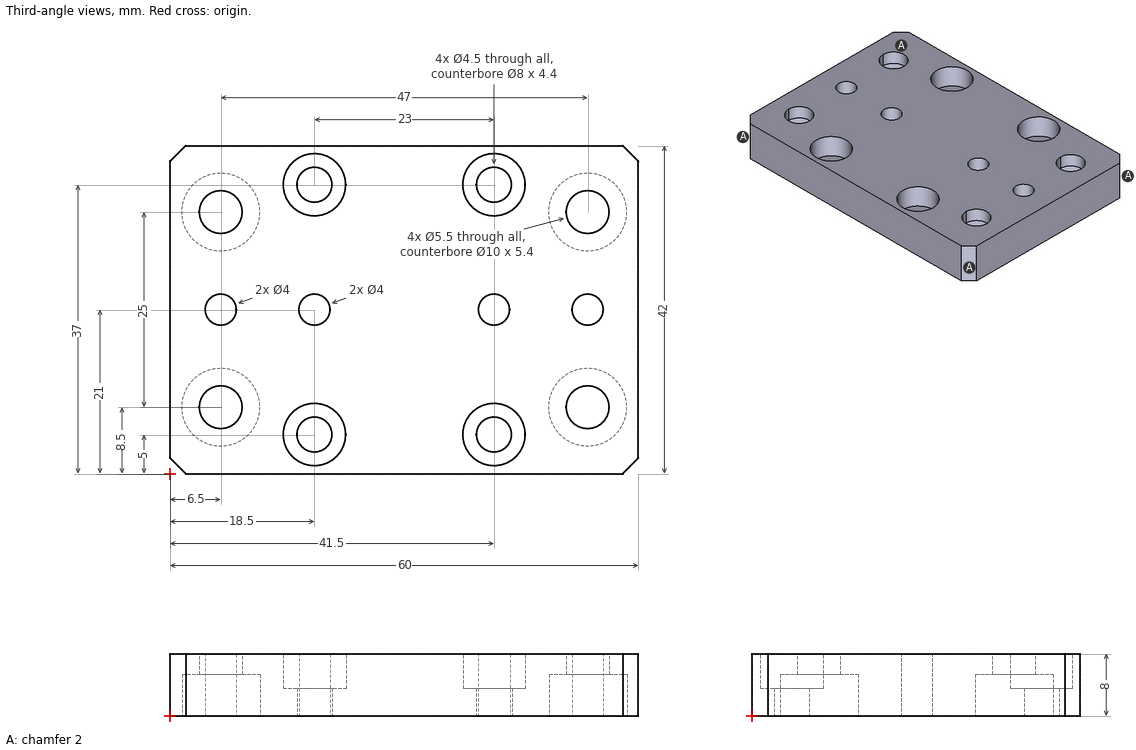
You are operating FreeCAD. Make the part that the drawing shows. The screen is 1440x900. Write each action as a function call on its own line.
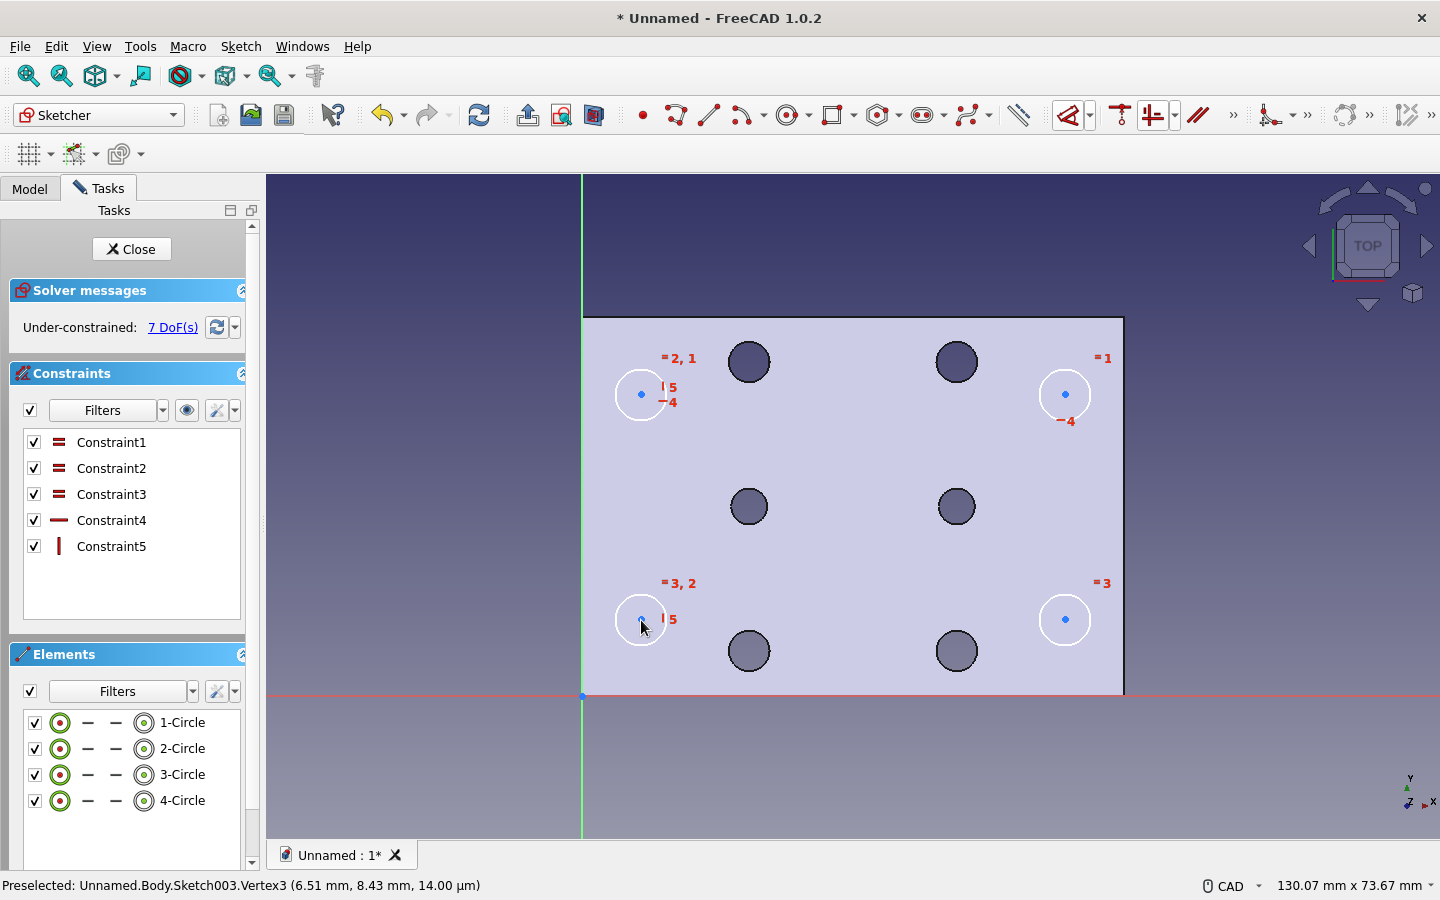
click(1065, 395)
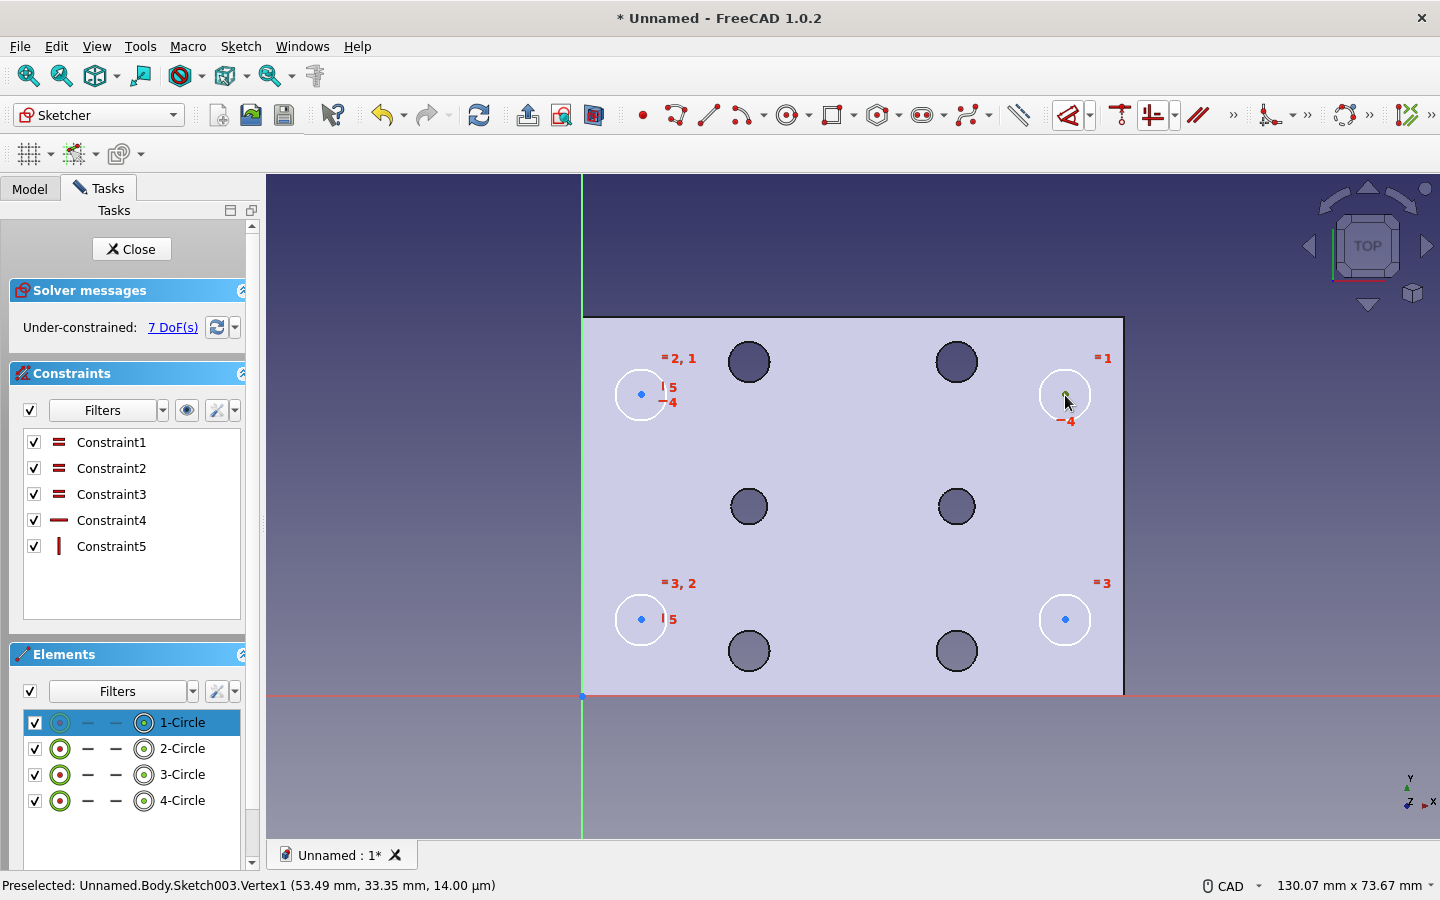
click(1065, 620)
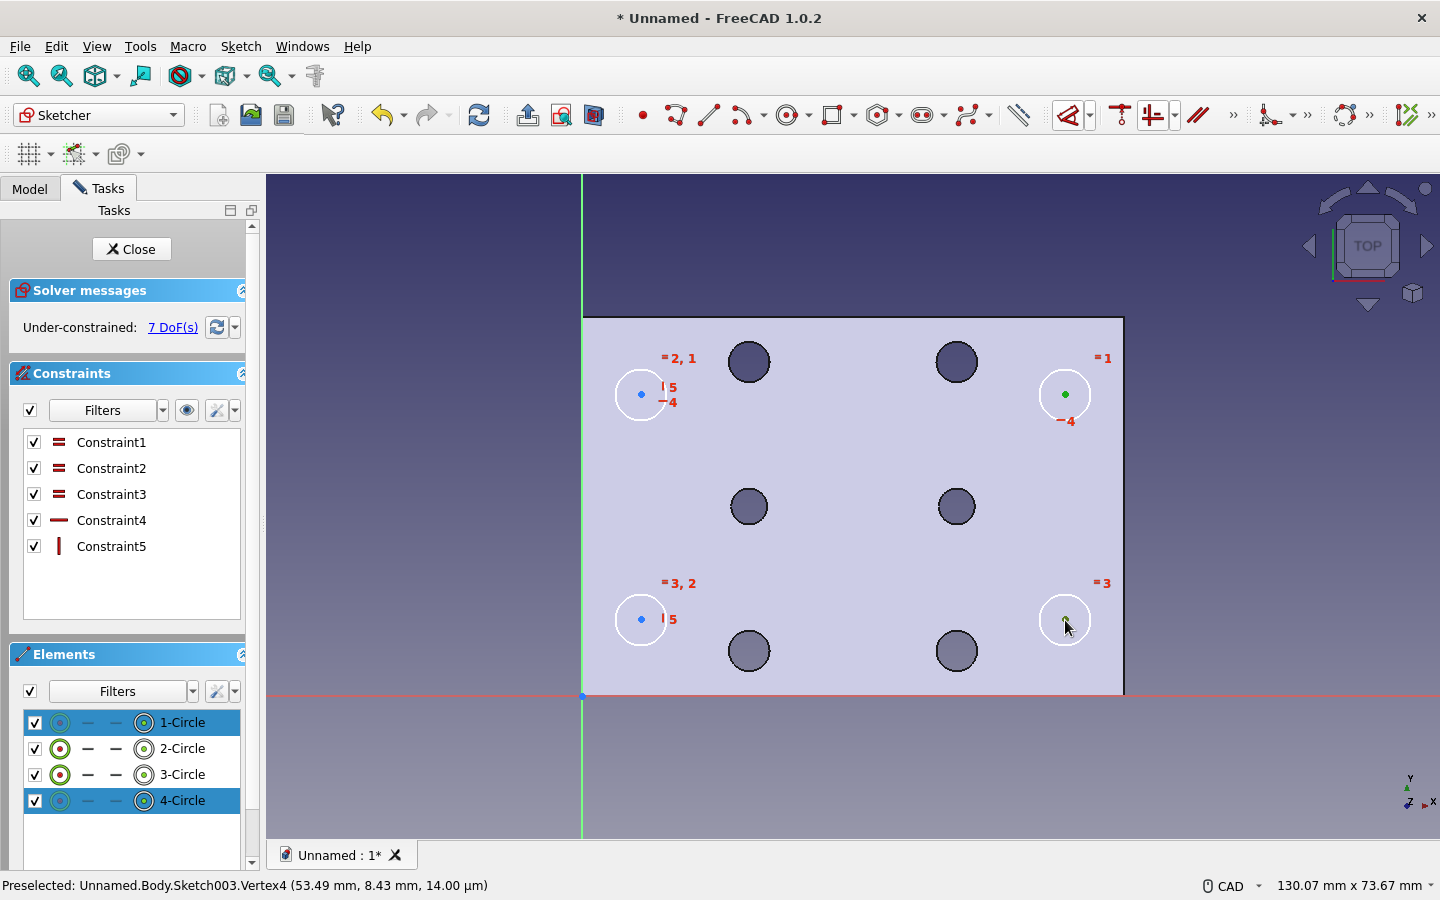
key(v)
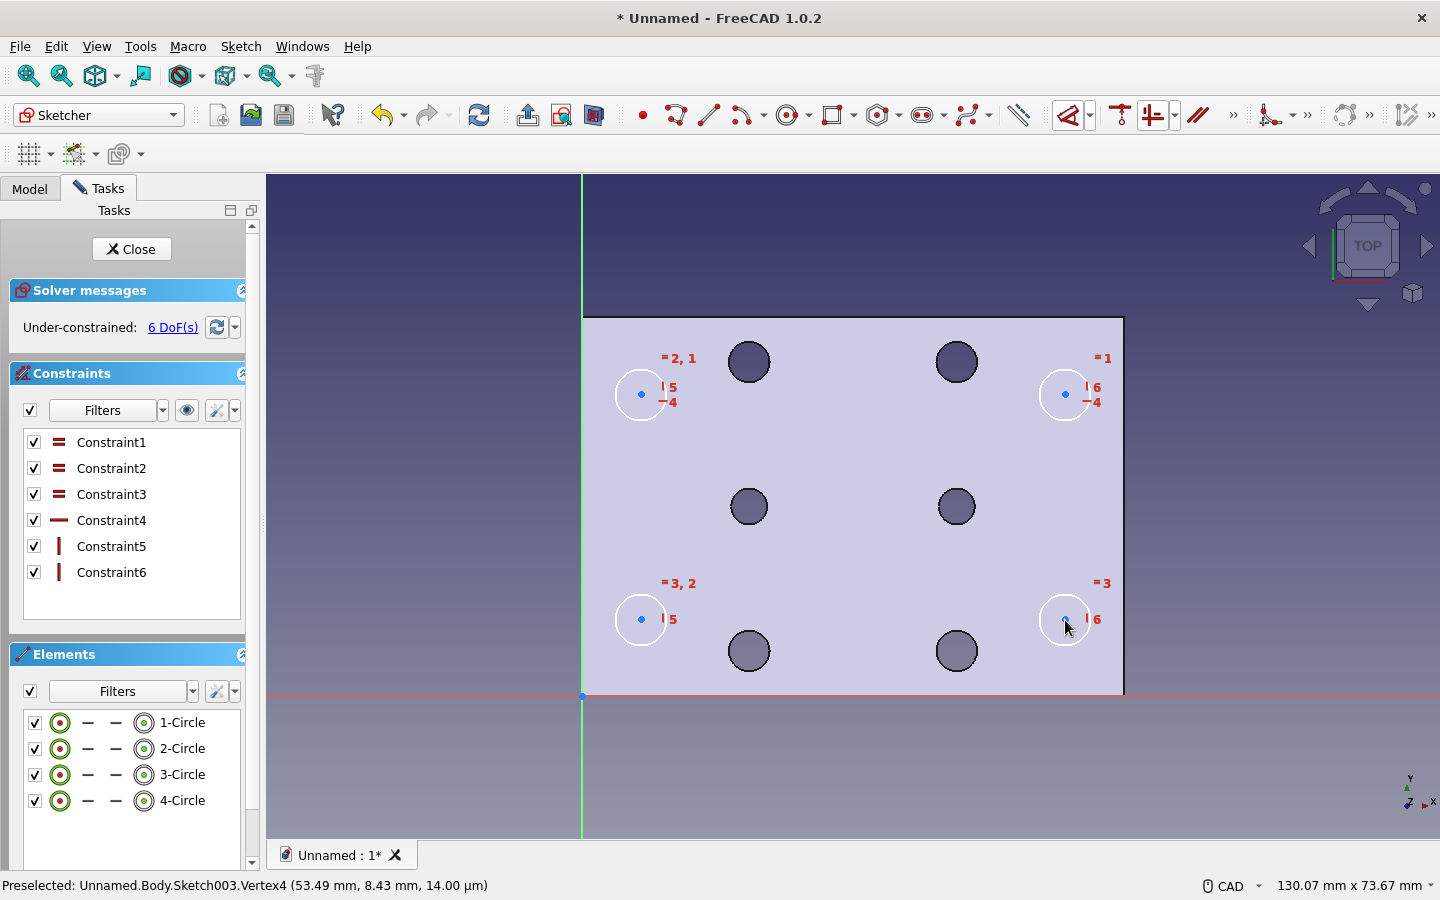
click(641, 620)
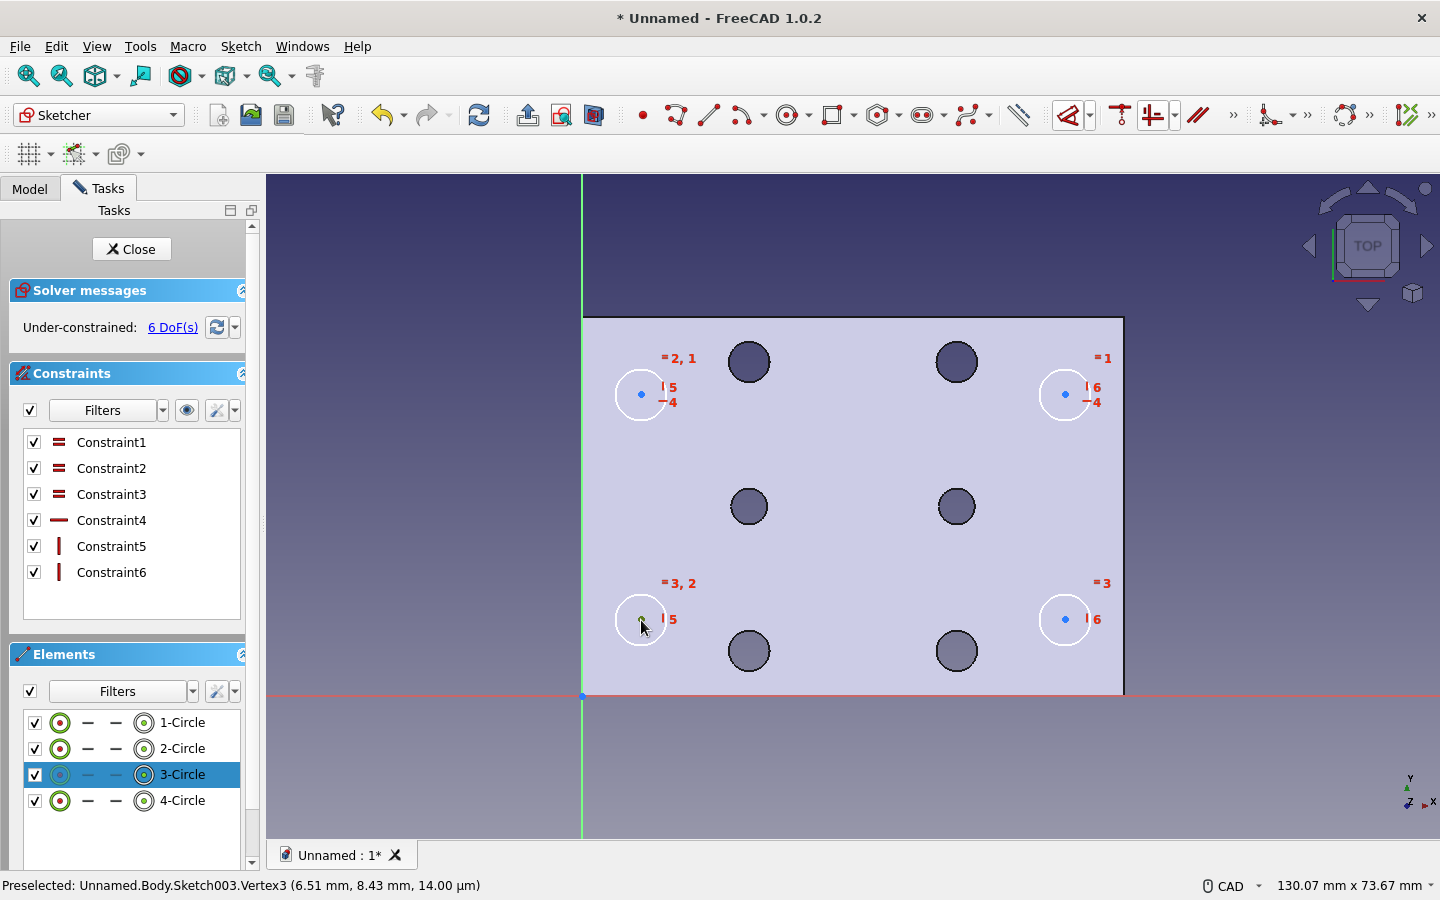
click(1065, 620)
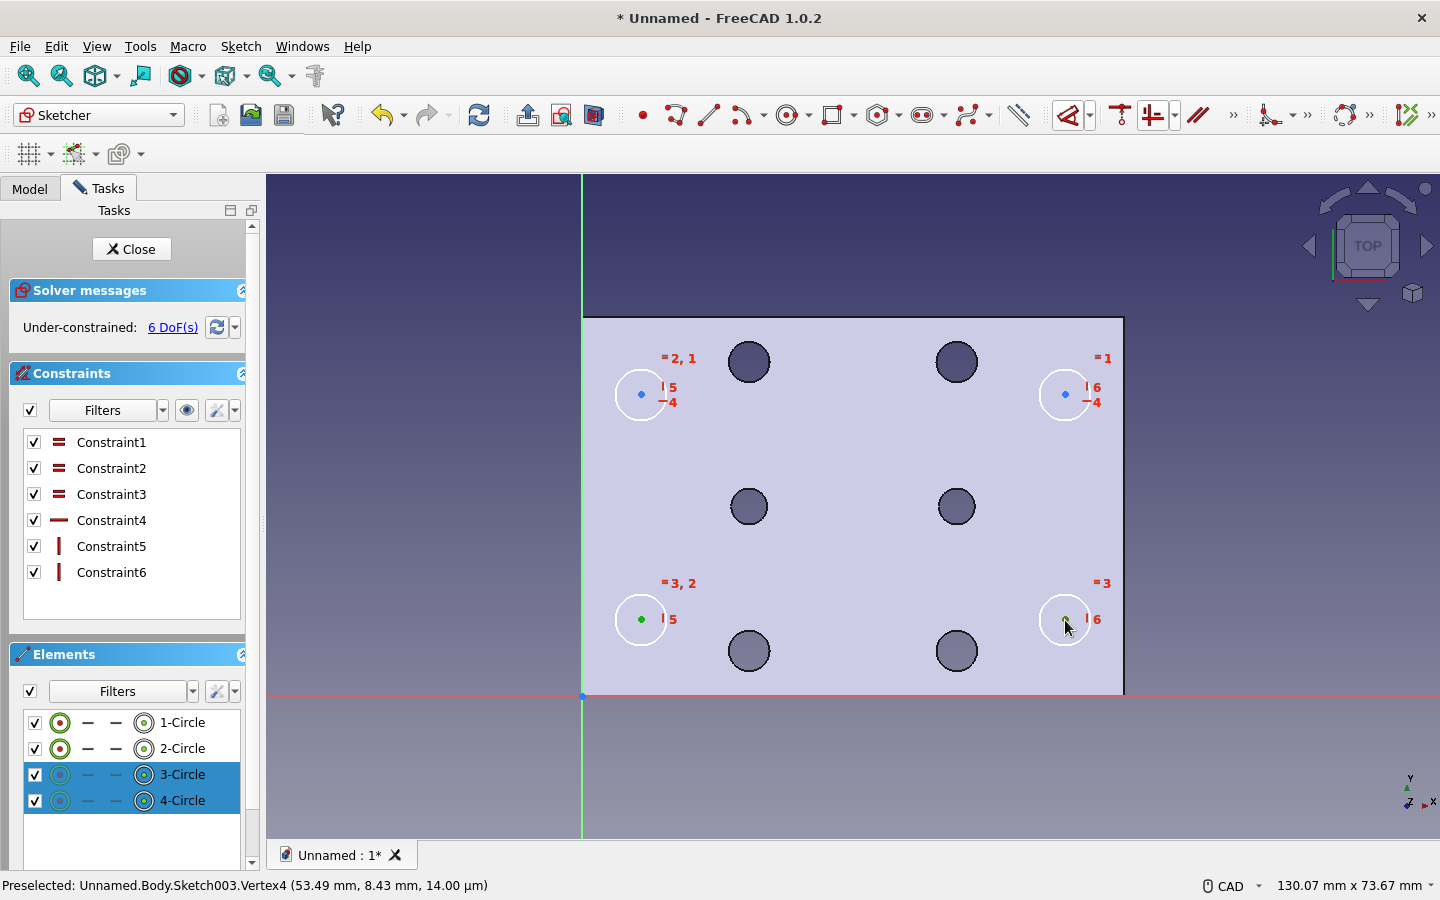
key(h)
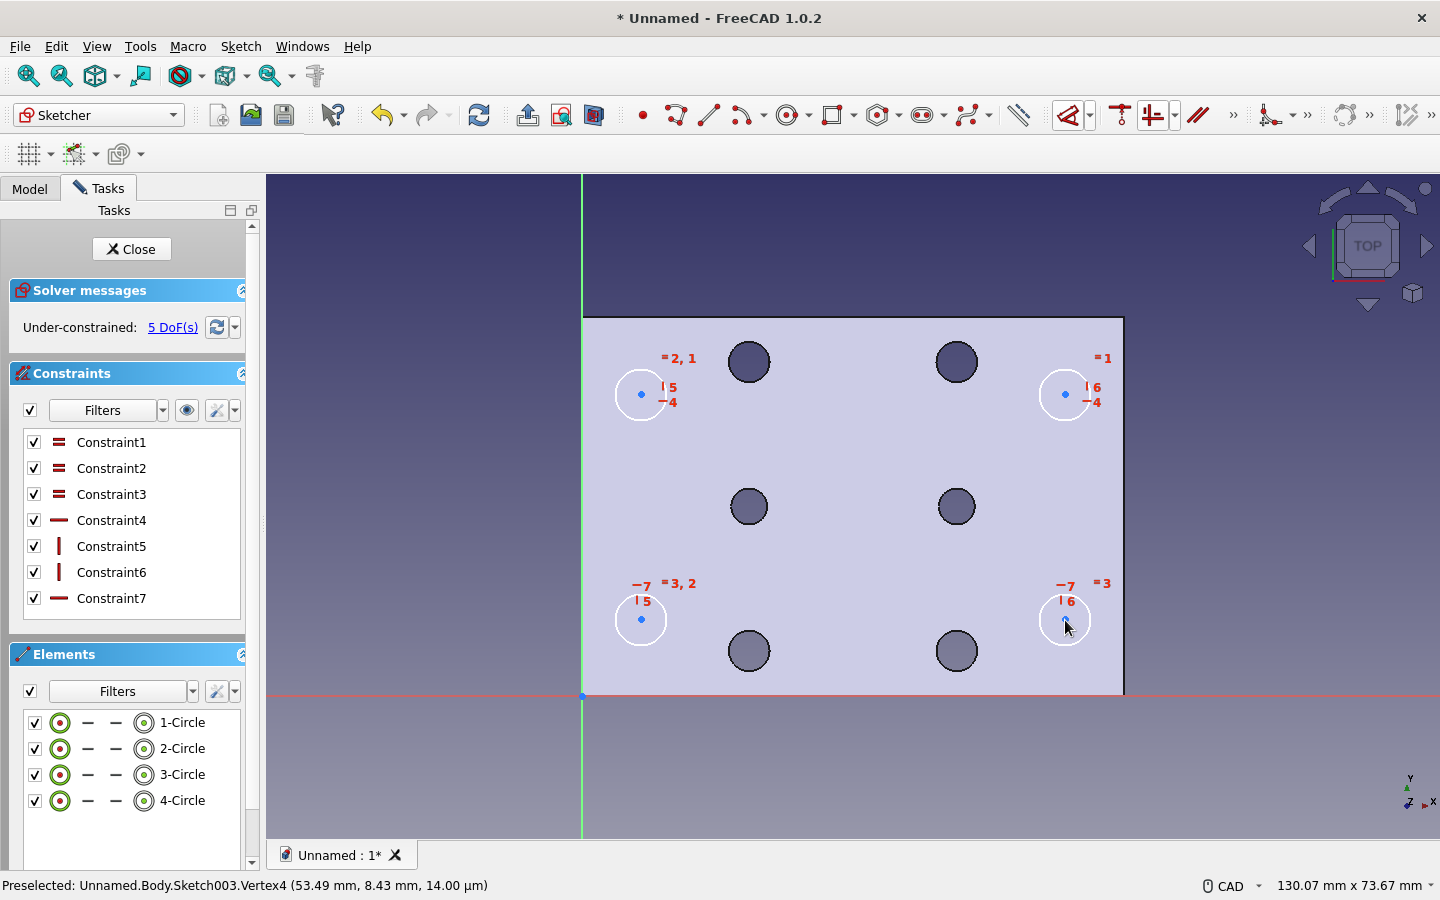
click(1083, 377)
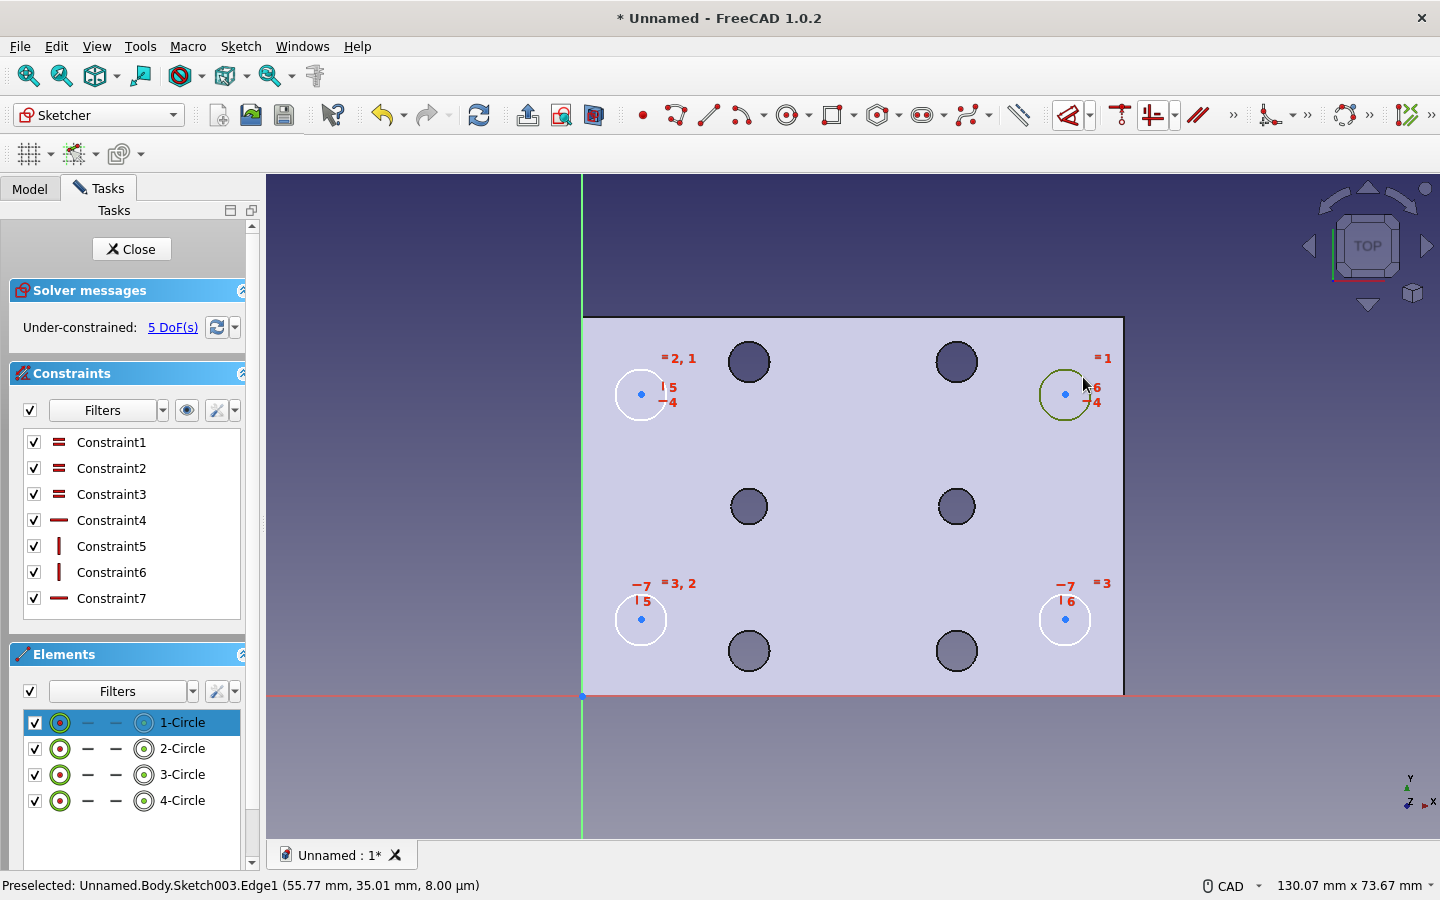
click(1090, 116)